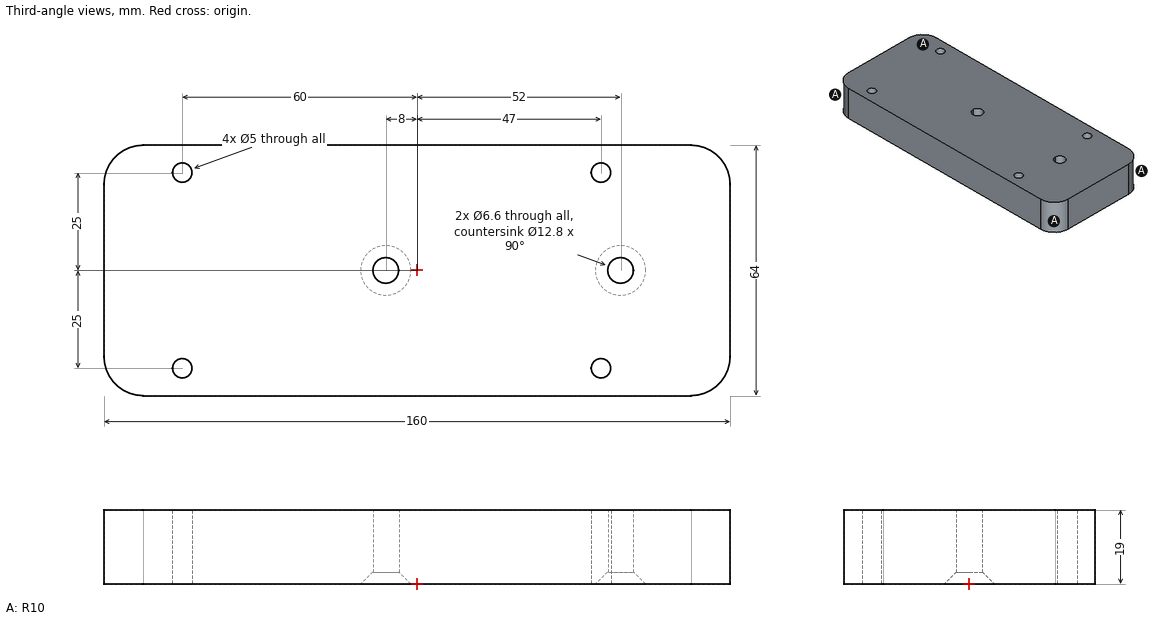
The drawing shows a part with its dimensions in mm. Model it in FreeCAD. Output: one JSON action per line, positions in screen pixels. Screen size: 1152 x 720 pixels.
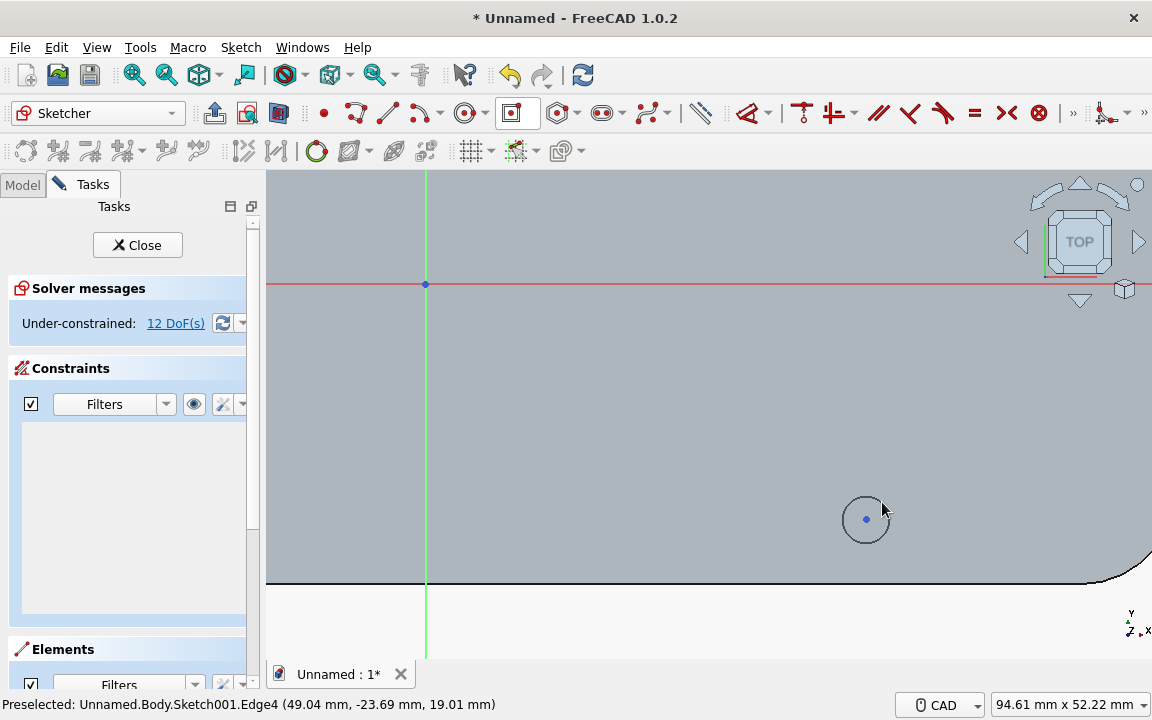
{"action": "scroll", "coordinate": [866, 521], "scroll_direction": "down", "scroll_amount": 4}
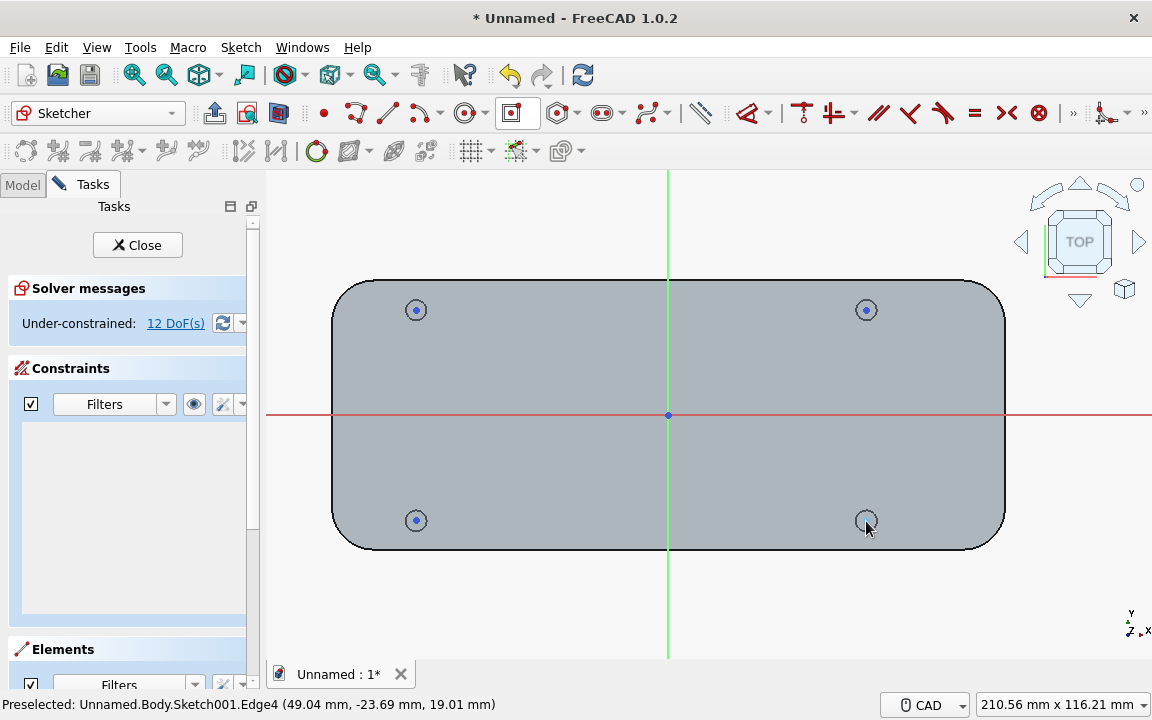
{"action": "scroll", "coordinate": [423, 303], "scroll_direction": "up", "scroll_amount": 2}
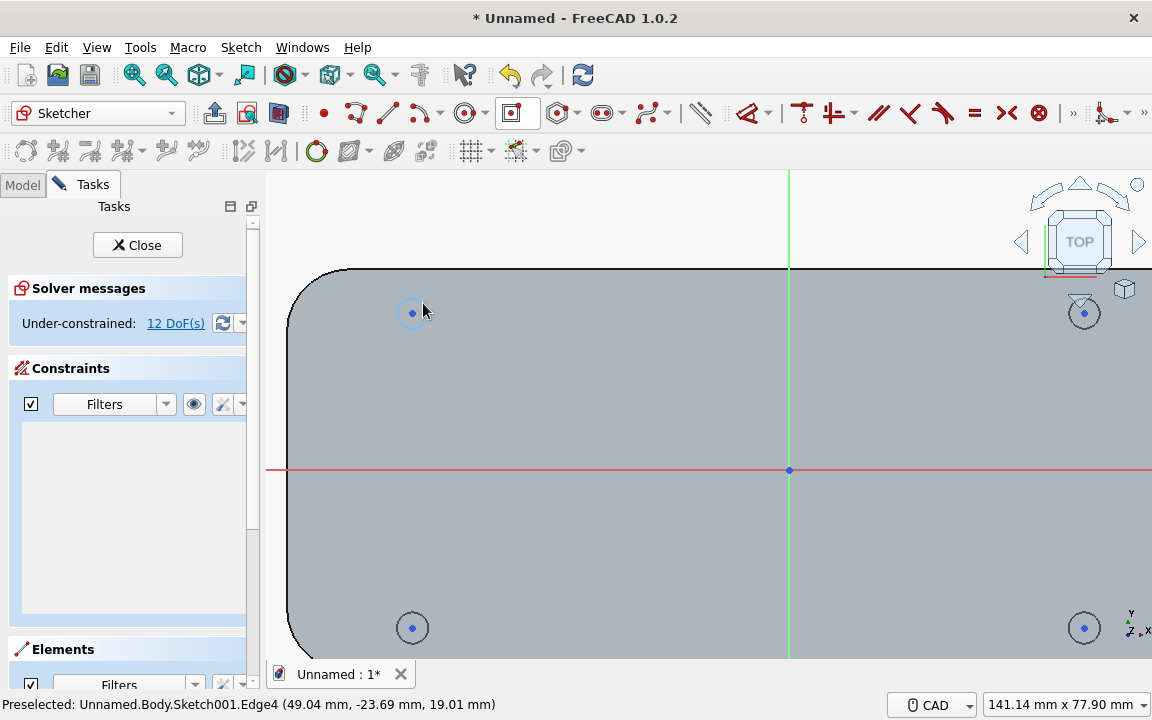
{"action": "left_click", "coordinate": [423, 303]}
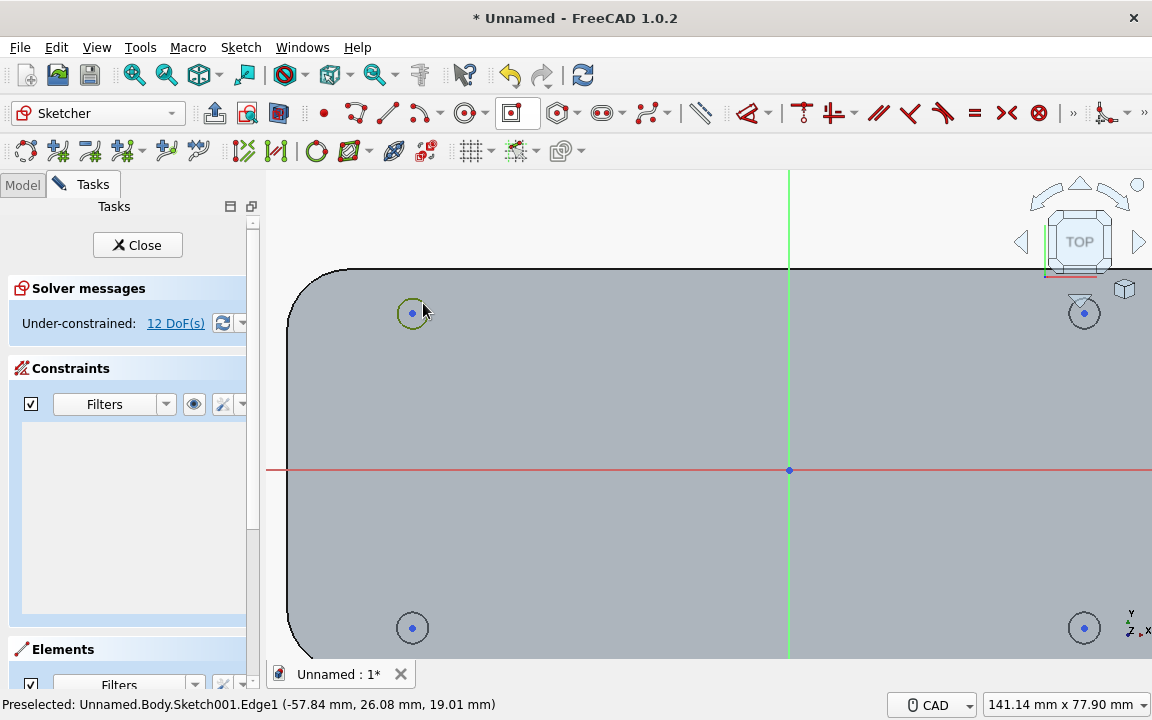
{"action": "left_click", "coordinate": [424, 617]}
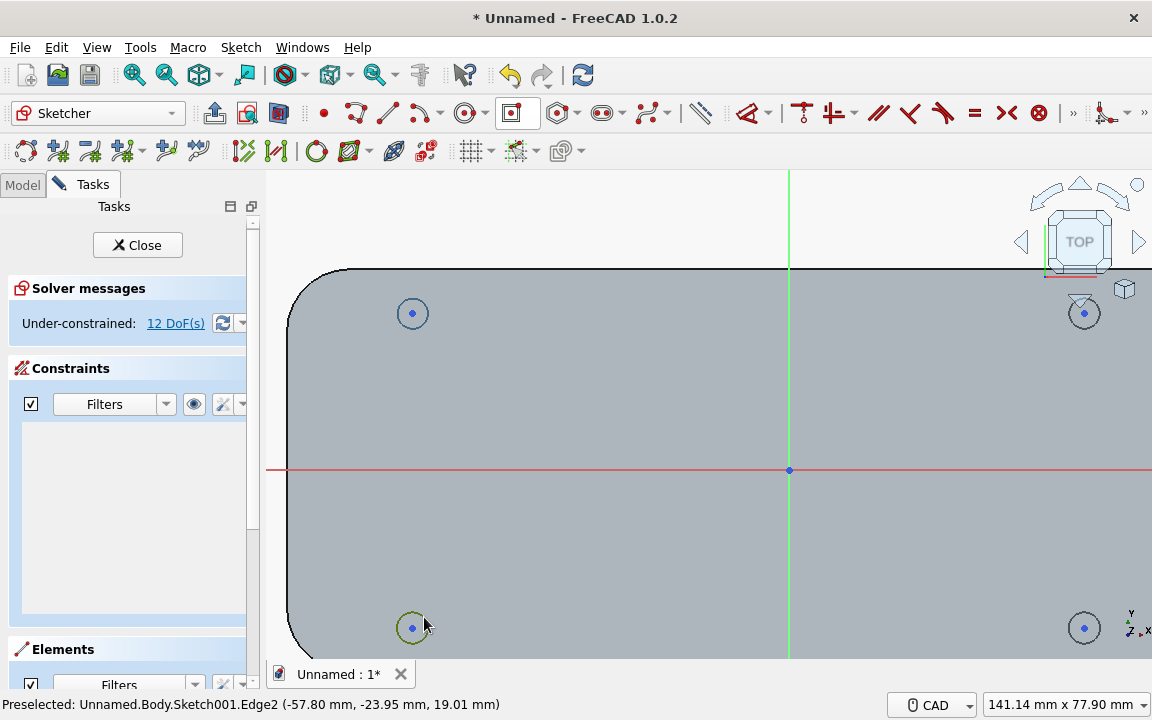
{"action": "scroll", "coordinate": [421, 301], "scroll_direction": "down", "scroll_amount": 2}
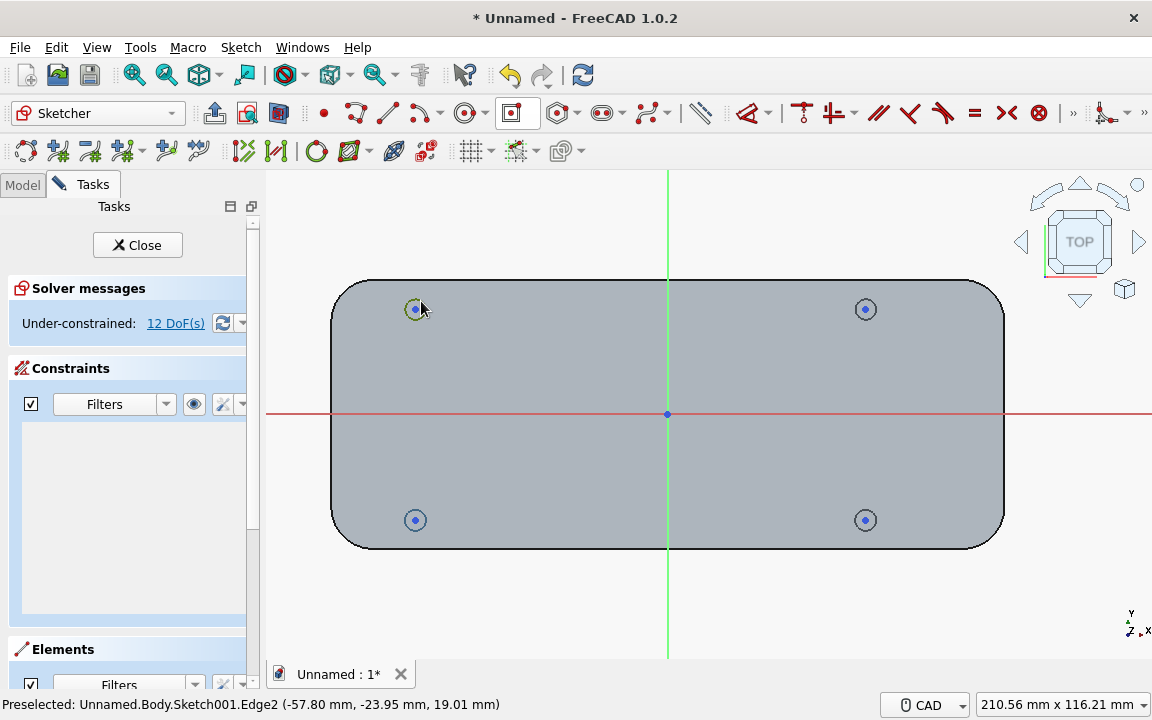
{"action": "scroll", "coordinate": [873, 302], "scroll_direction": "up", "scroll_amount": 2}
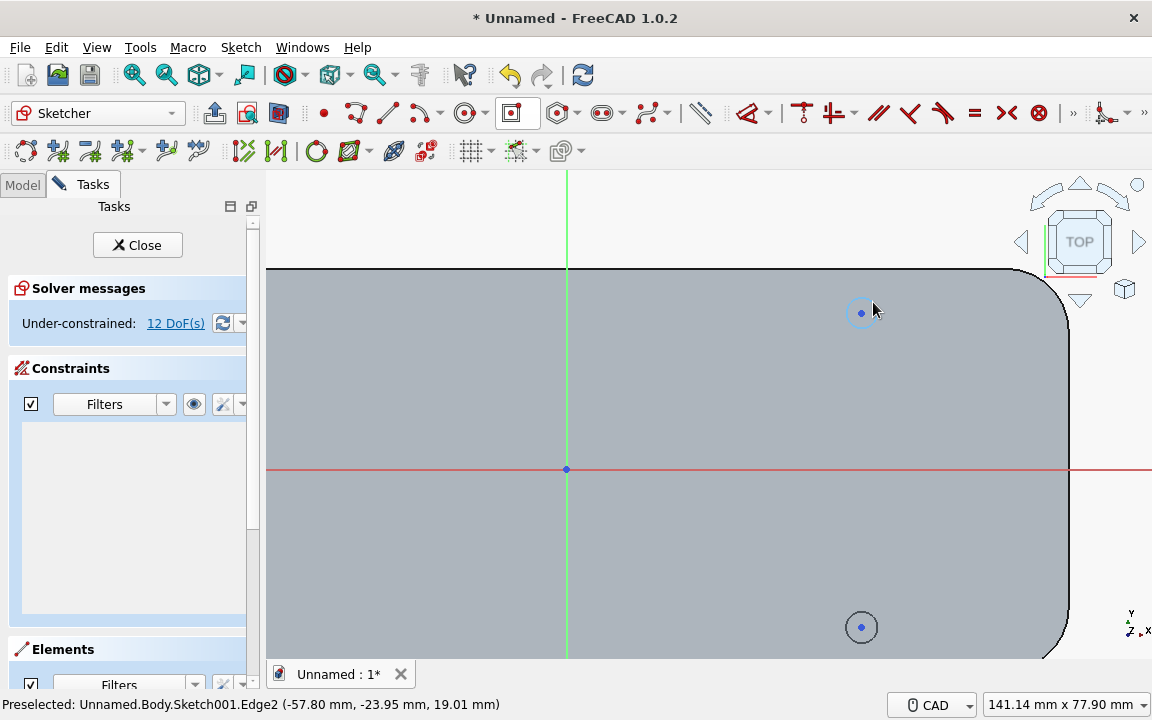
{"action": "left_click", "coordinate": [873, 302]}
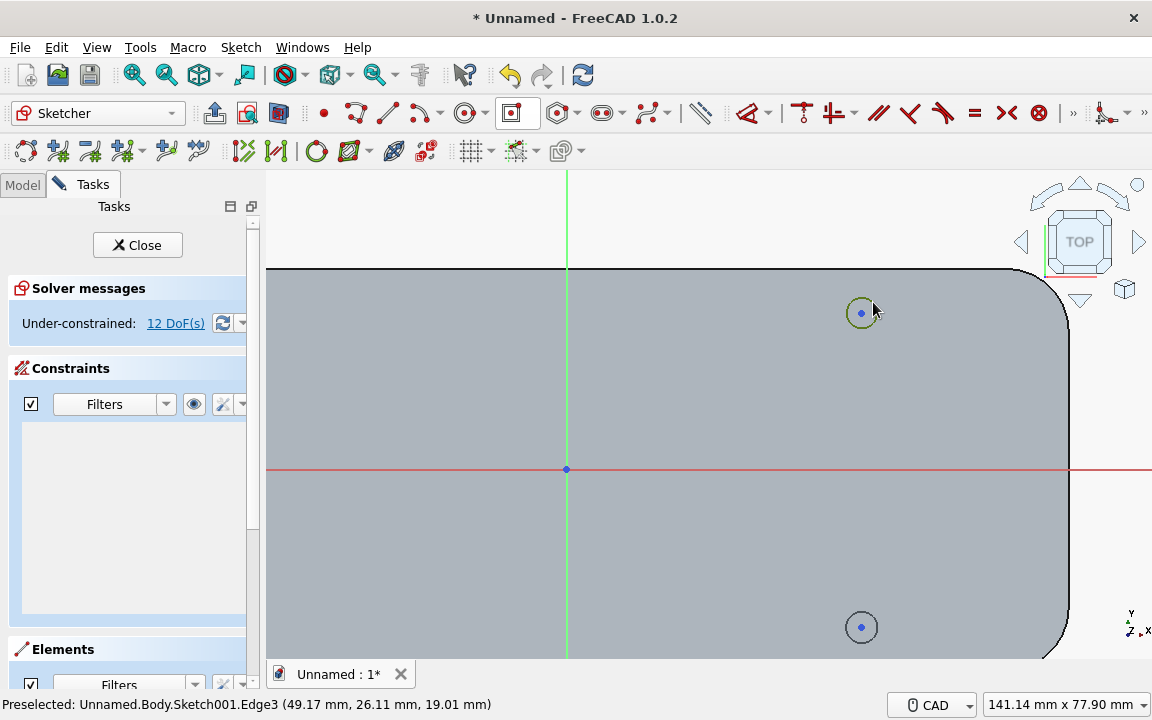
{"action": "left_click", "coordinate": [873, 616]}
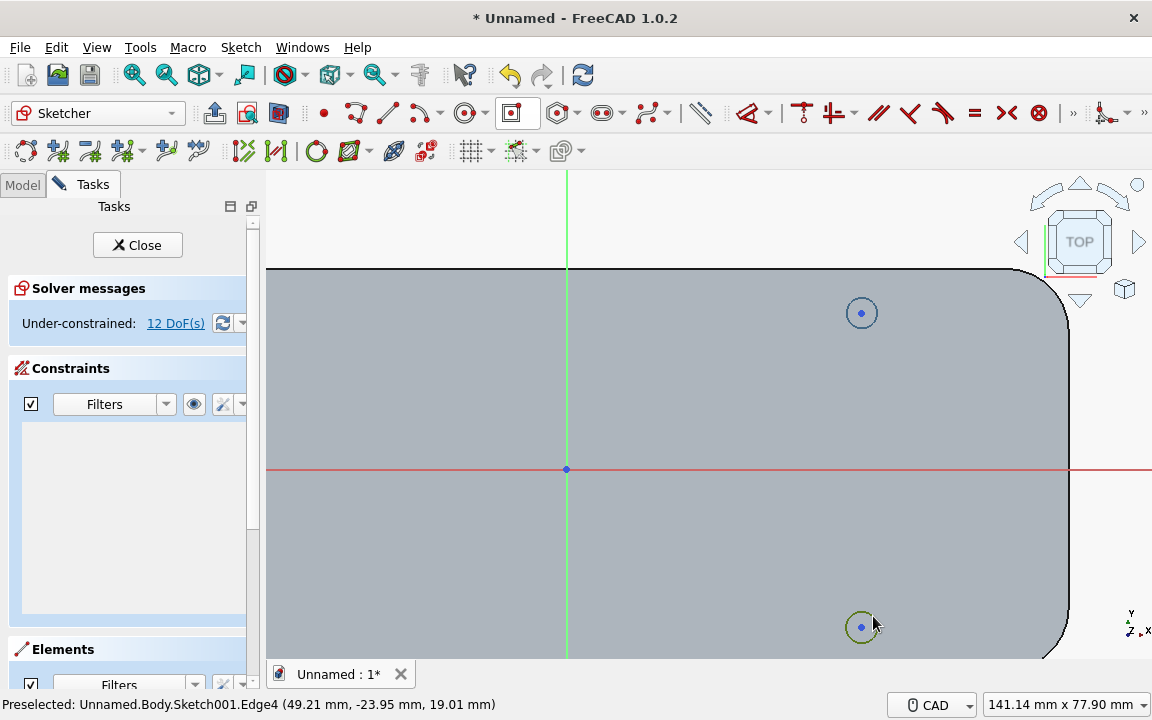
{"action": "left_click", "coordinate": [976, 114]}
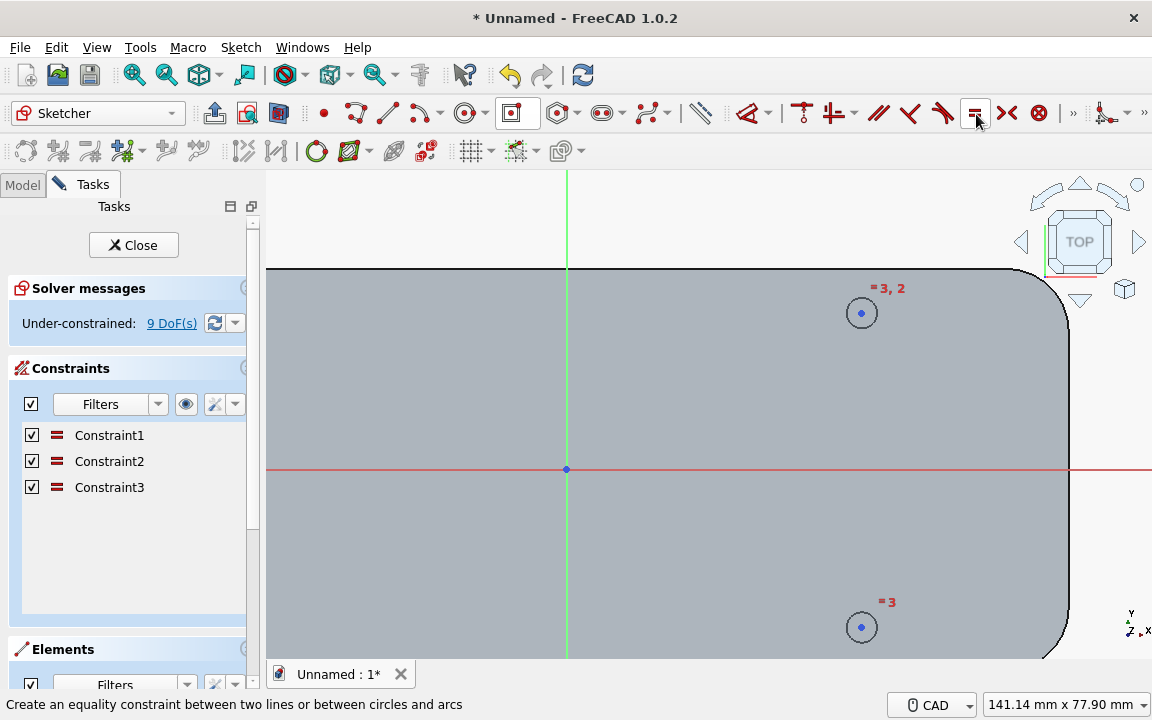
{"action": "scroll", "coordinate": [874, 302], "scroll_direction": "down", "scroll_amount": 2}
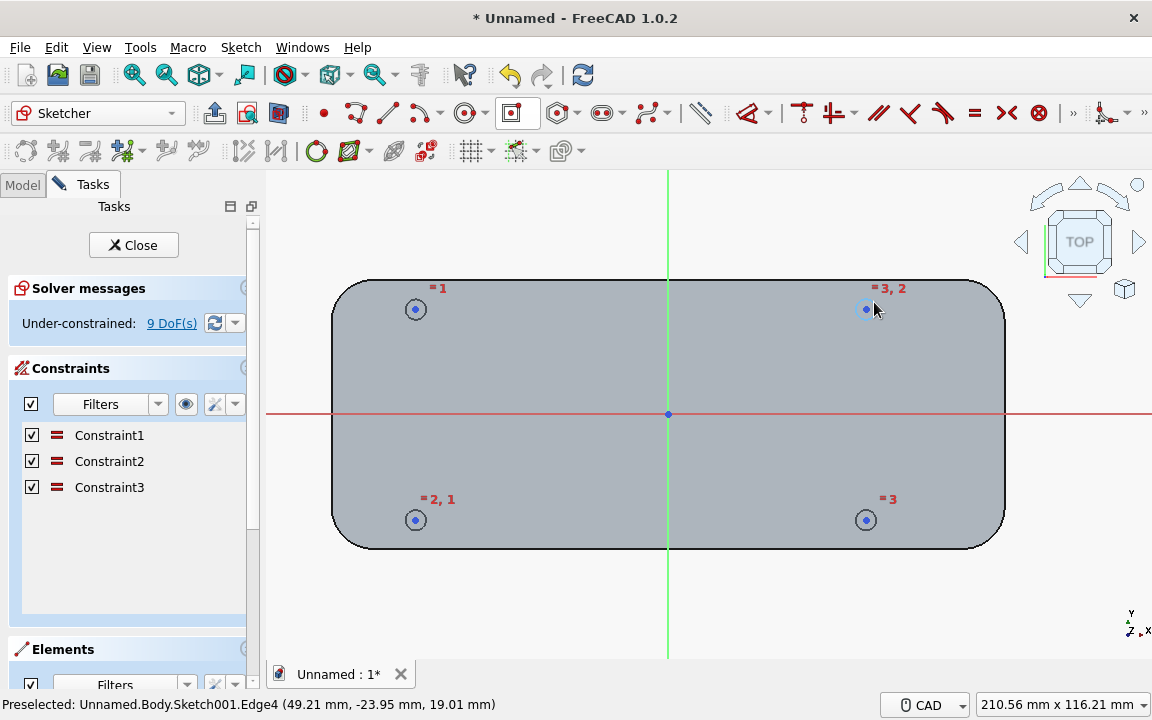
{"action": "left_click", "coordinate": [416, 310]}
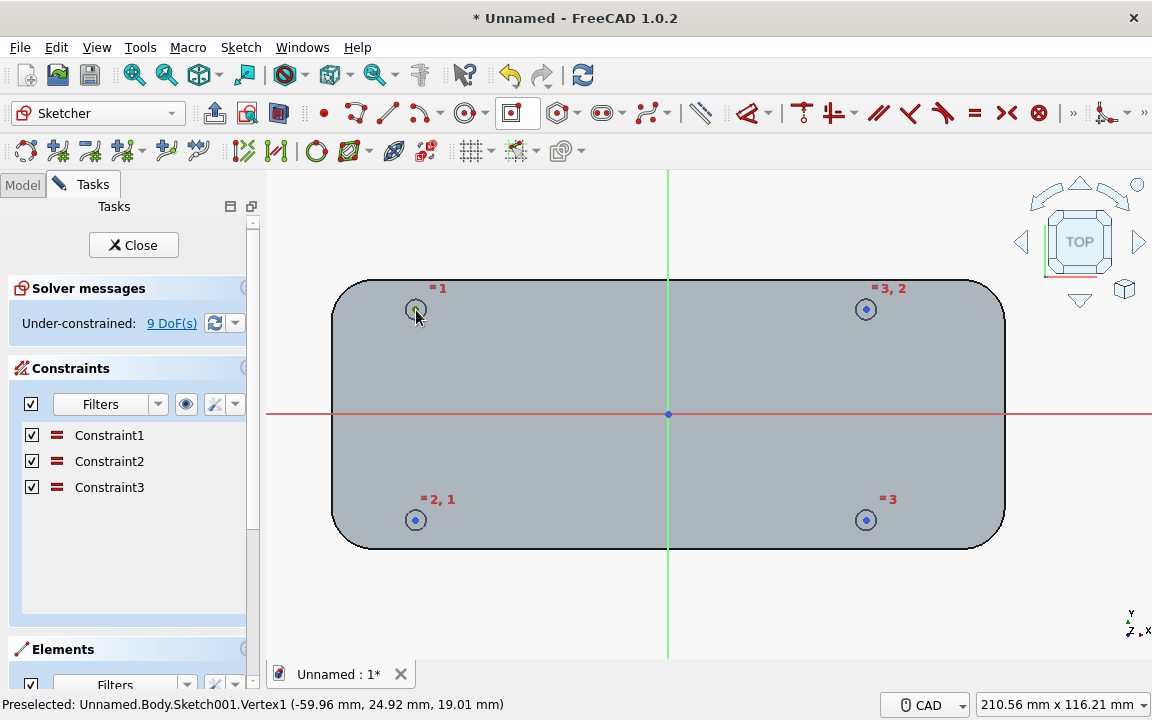
{"action": "left_click", "coordinate": [416, 520]}